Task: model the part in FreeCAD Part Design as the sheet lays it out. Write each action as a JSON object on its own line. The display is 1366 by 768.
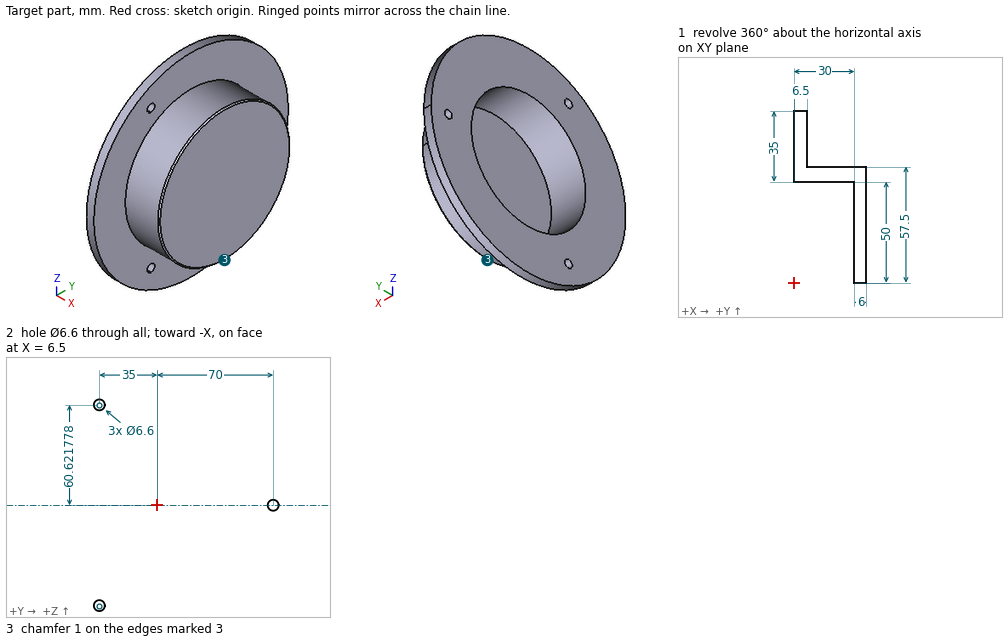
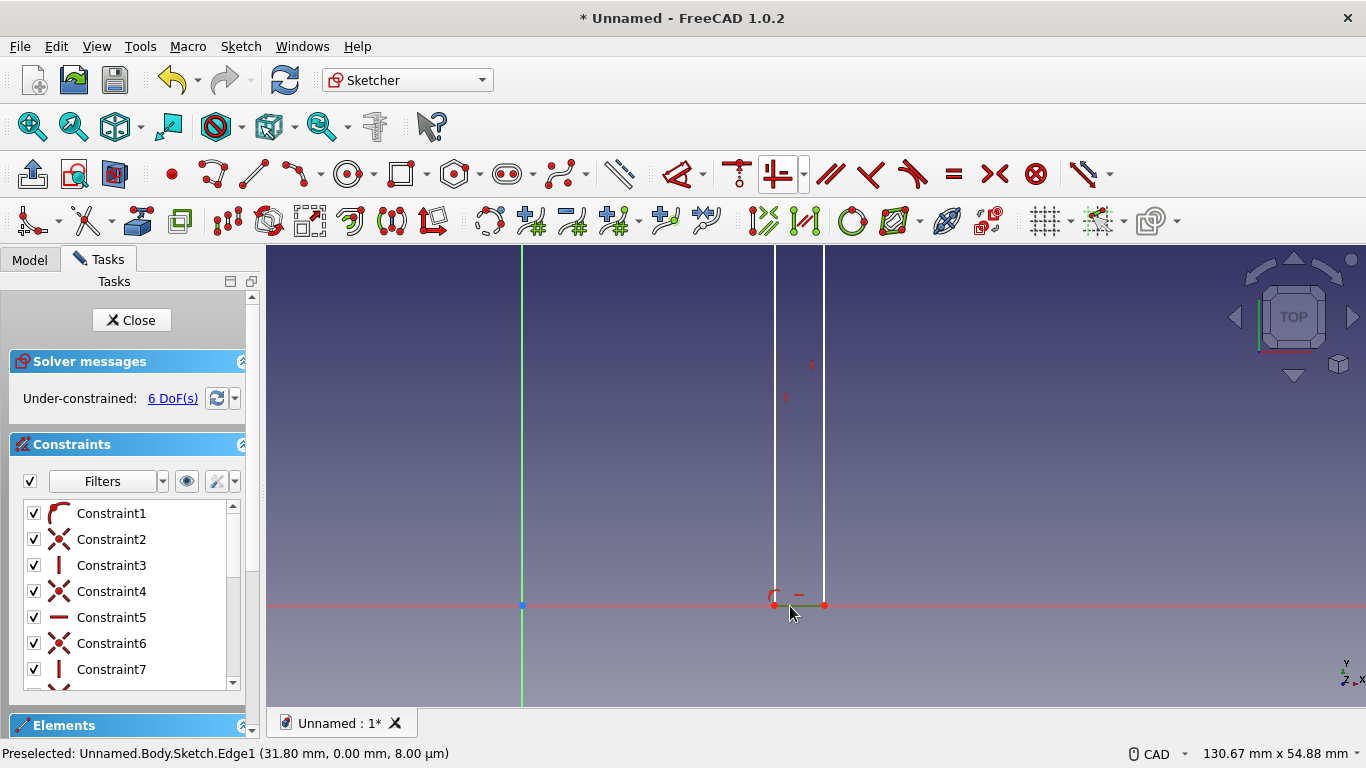
{"action": "left_click", "coordinate": [702, 174]}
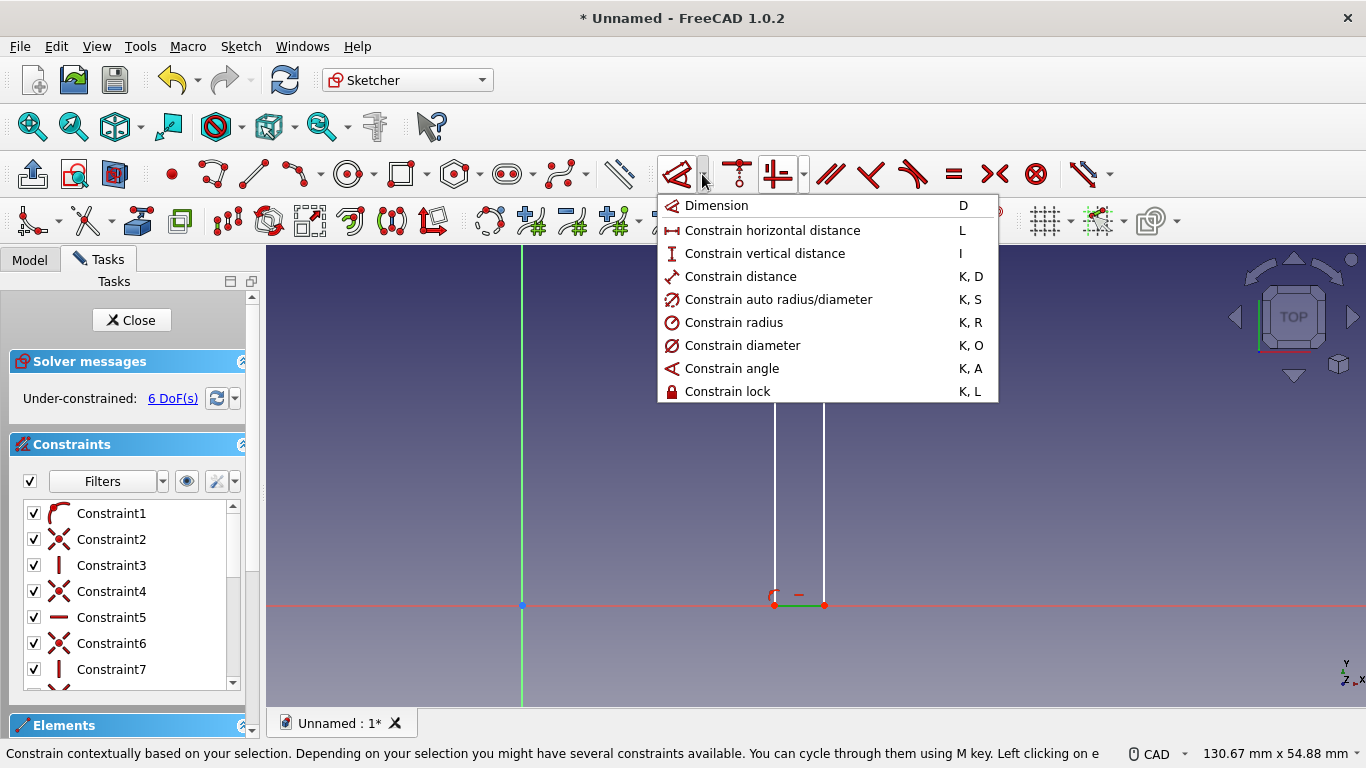
{"action": "left_click", "coordinate": [828, 230]}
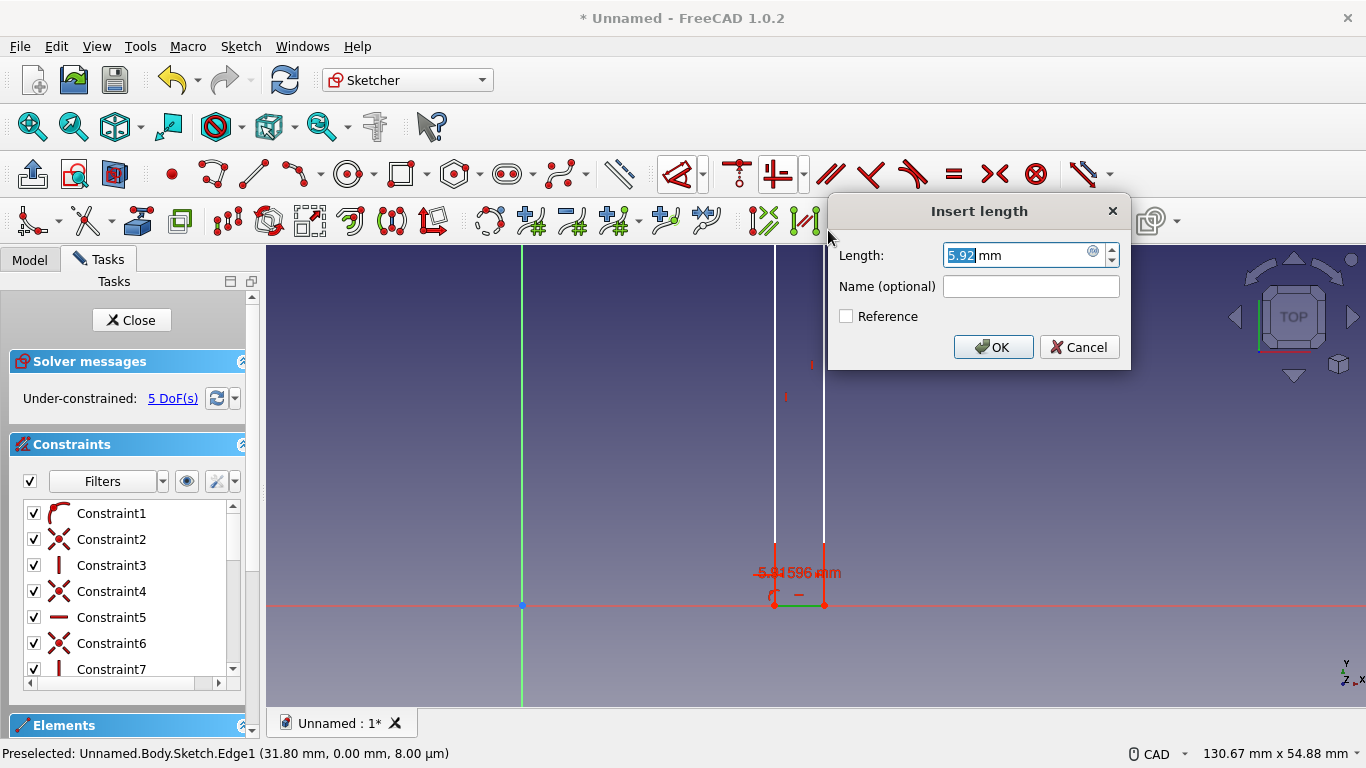
{"action": "type", "text": "6"}
{"action": "key", "text": "Return"}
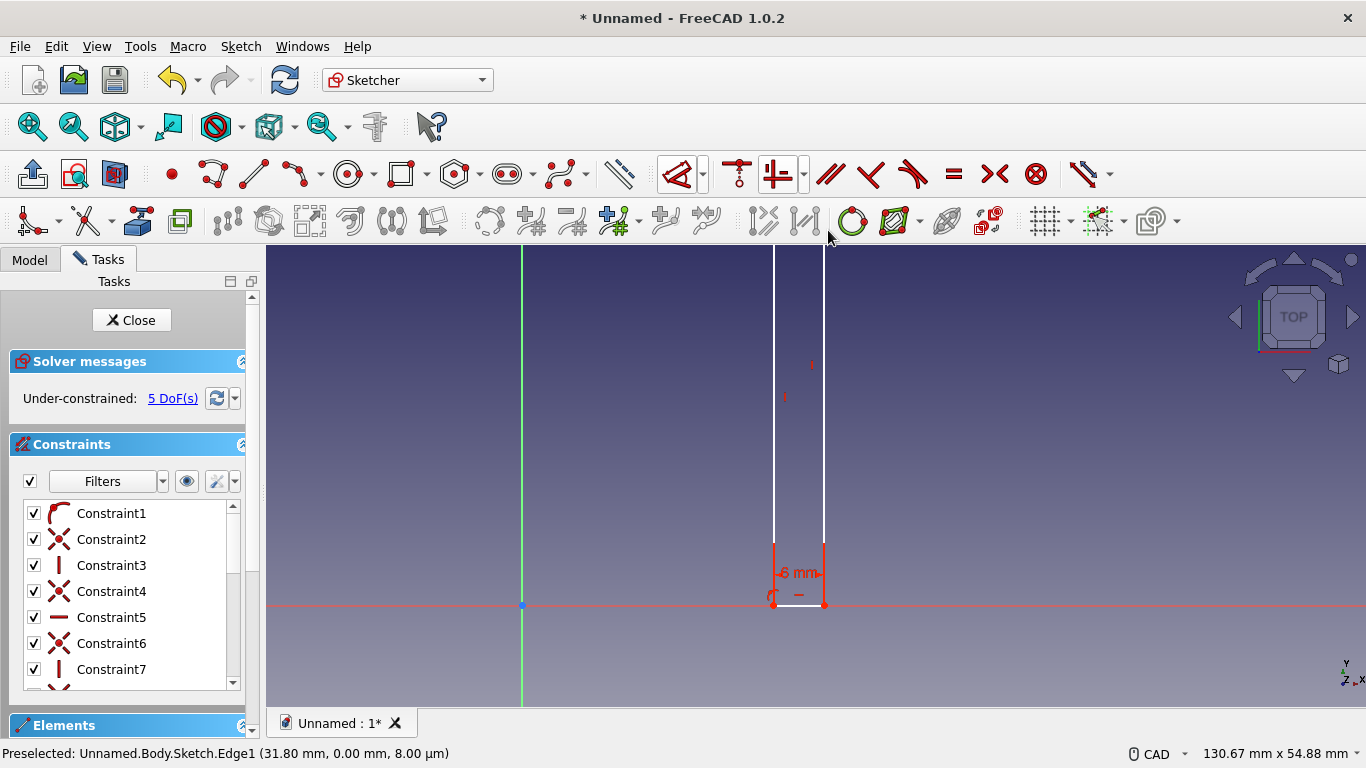
{"action": "scroll", "coordinate": [790, 609], "scroll_direction": "down", "scroll_amount": 5}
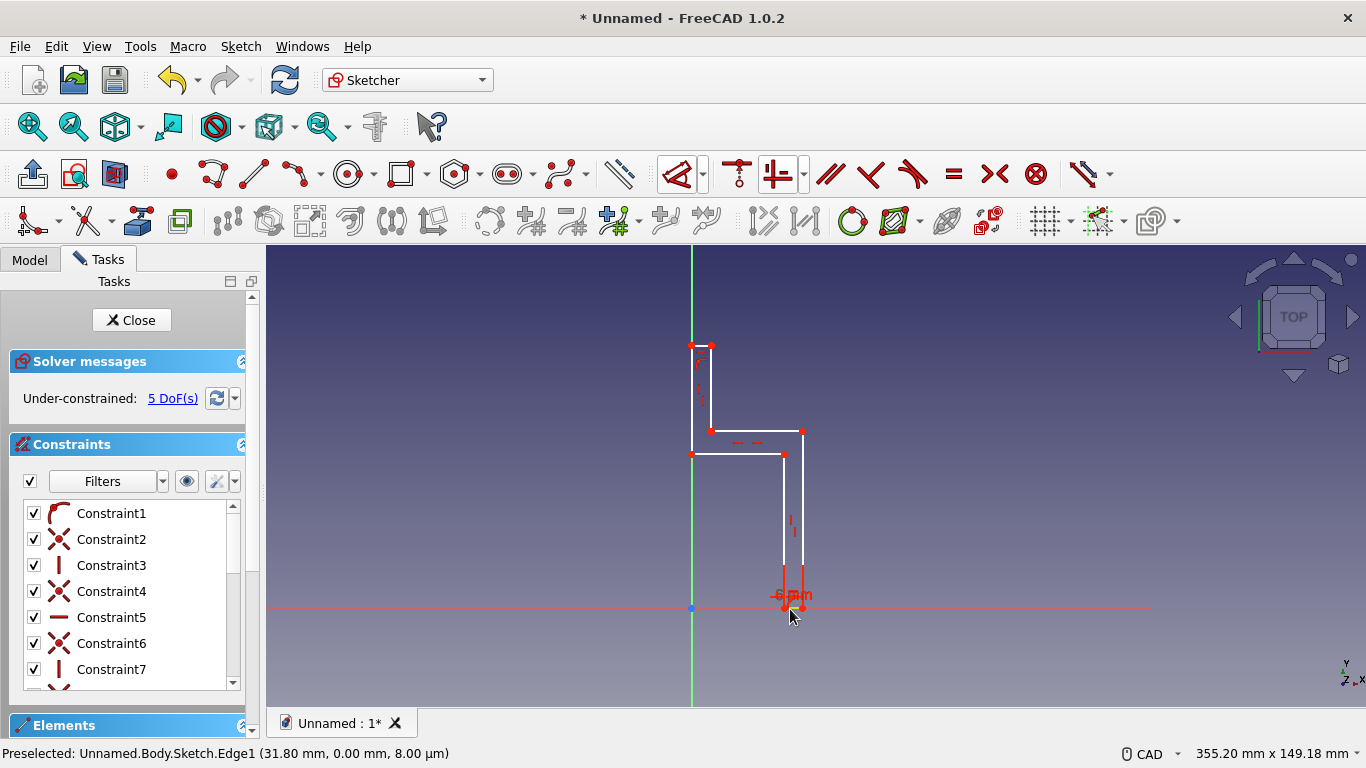
{"action": "left_click", "coordinate": [692, 378]}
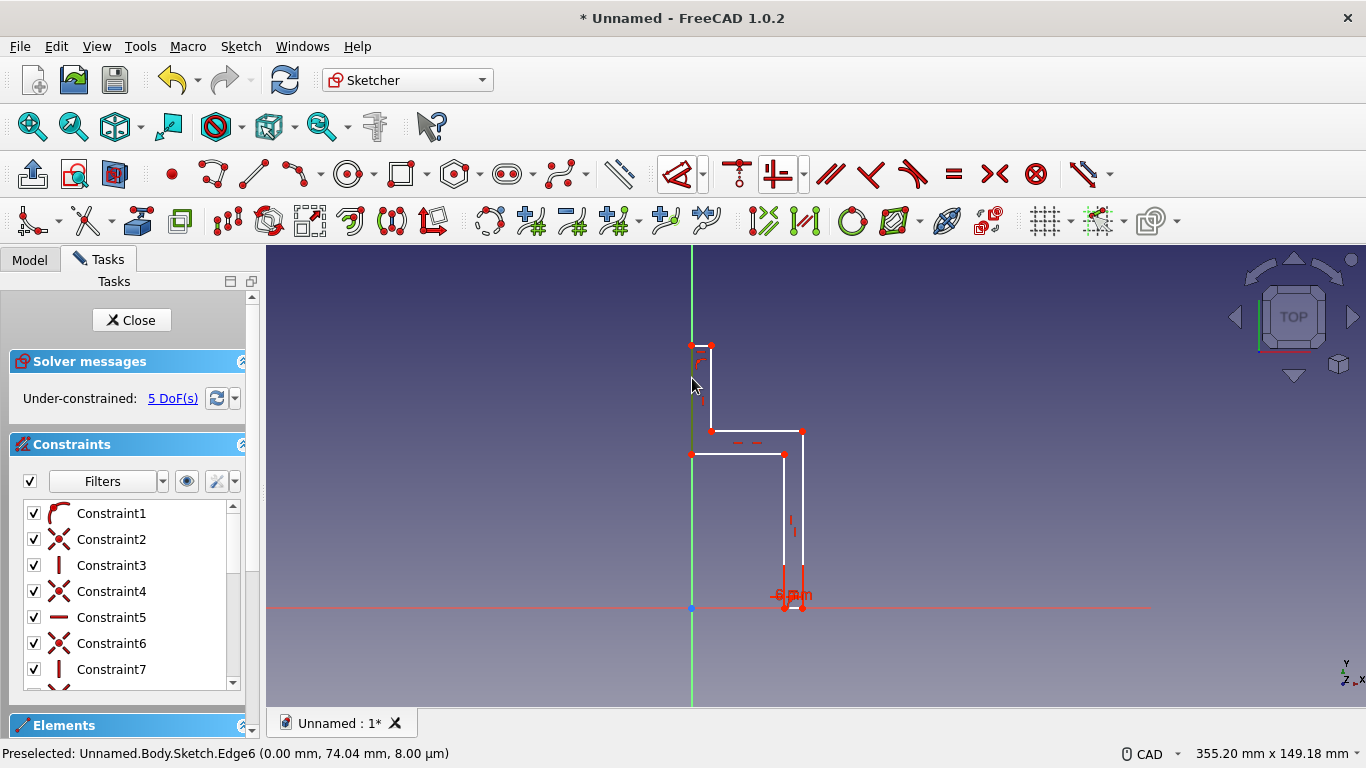
{"action": "left_click", "coordinate": [702, 174]}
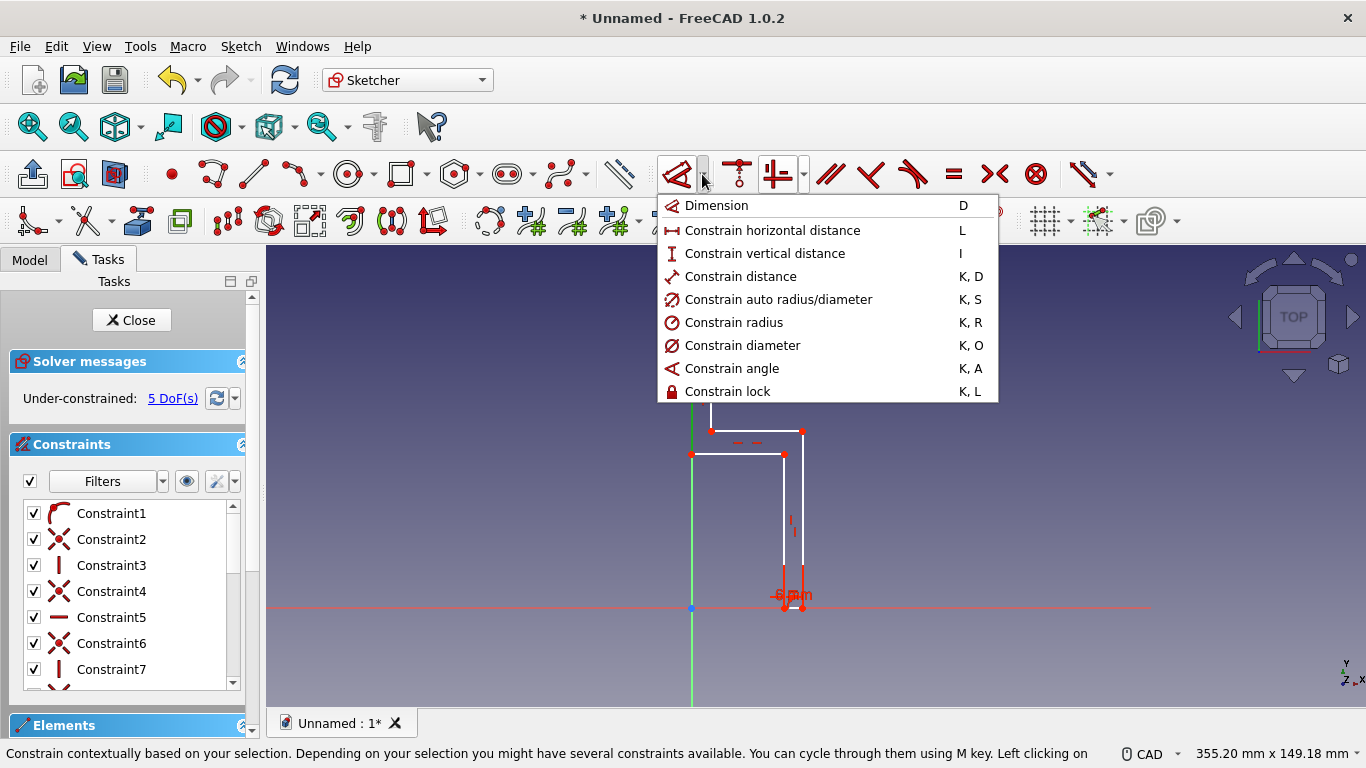
{"action": "left_click", "coordinate": [828, 254]}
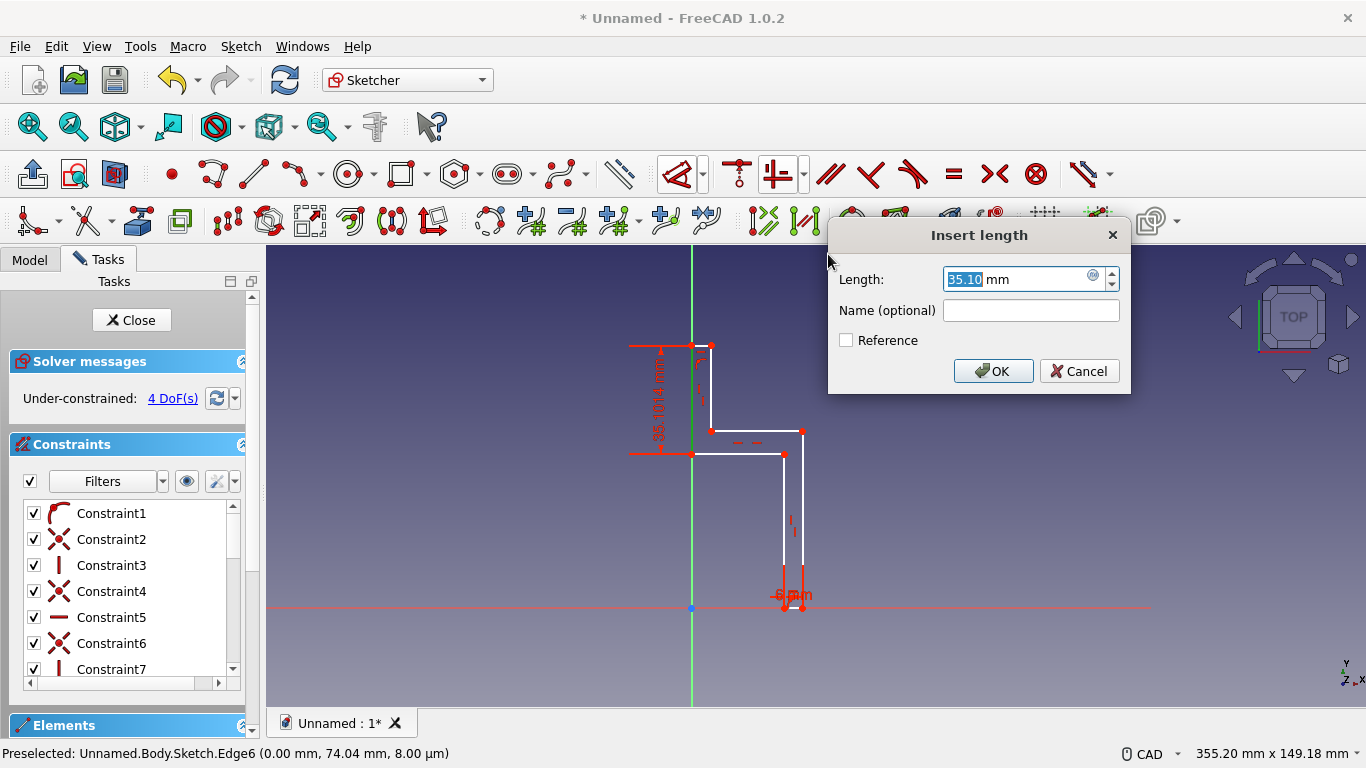
{"action": "type", "text": "35"}
{"action": "key", "text": "Return"}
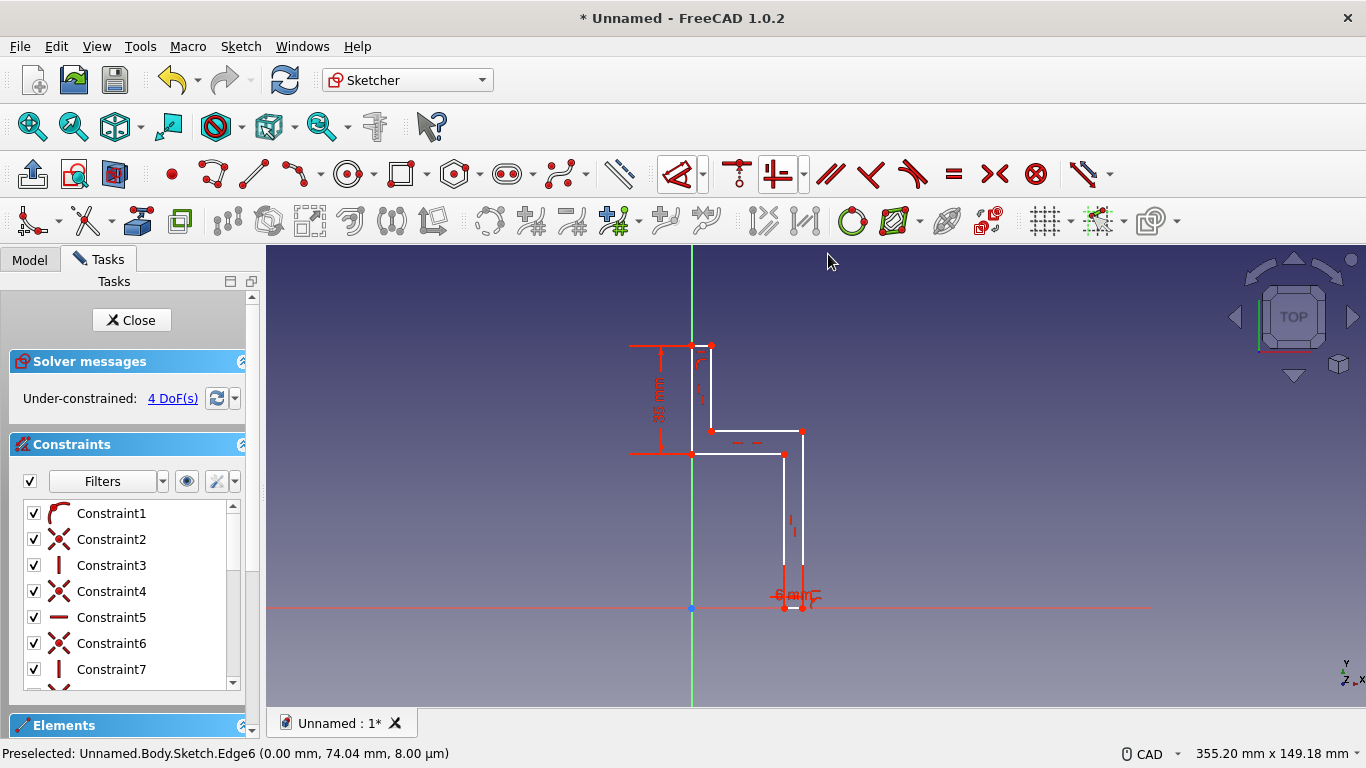
{"action": "left_click", "coordinate": [720, 454]}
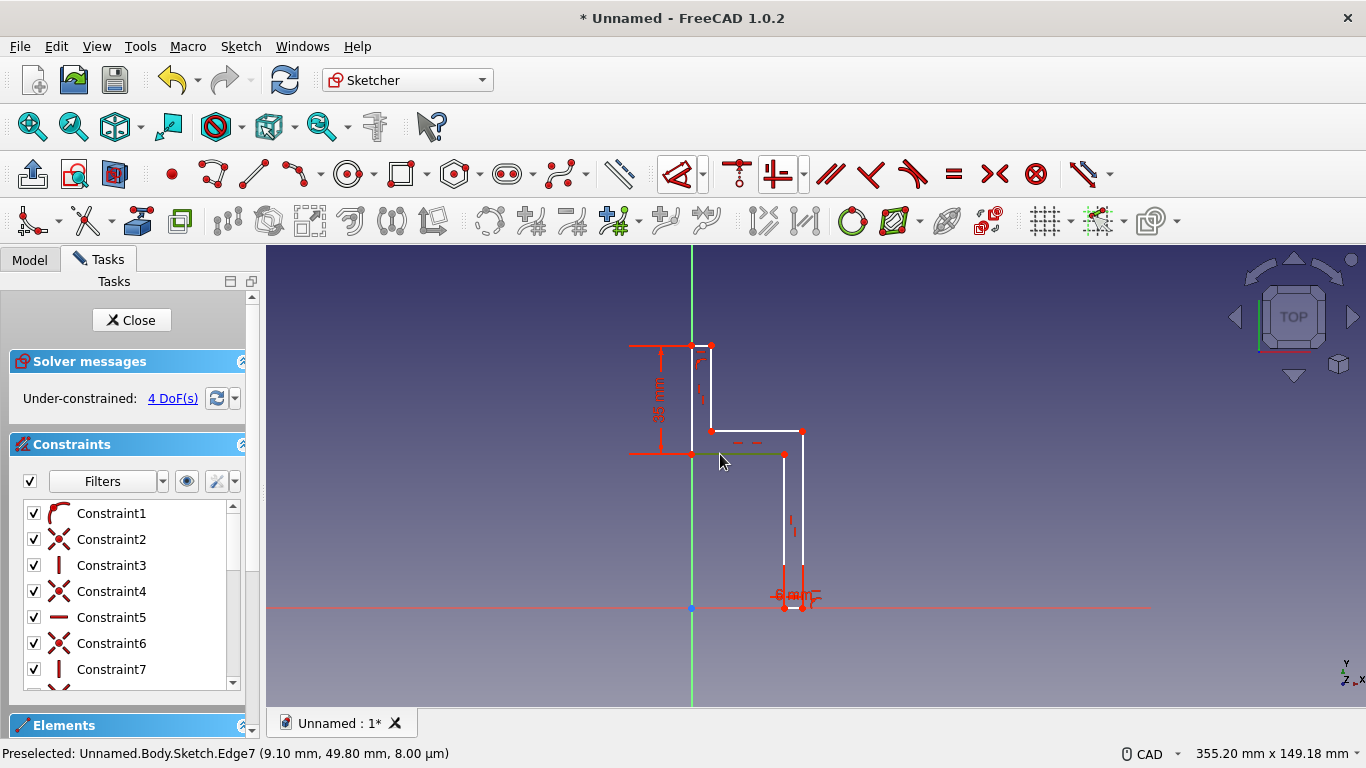
{"action": "left_click", "coordinate": [702, 174]}